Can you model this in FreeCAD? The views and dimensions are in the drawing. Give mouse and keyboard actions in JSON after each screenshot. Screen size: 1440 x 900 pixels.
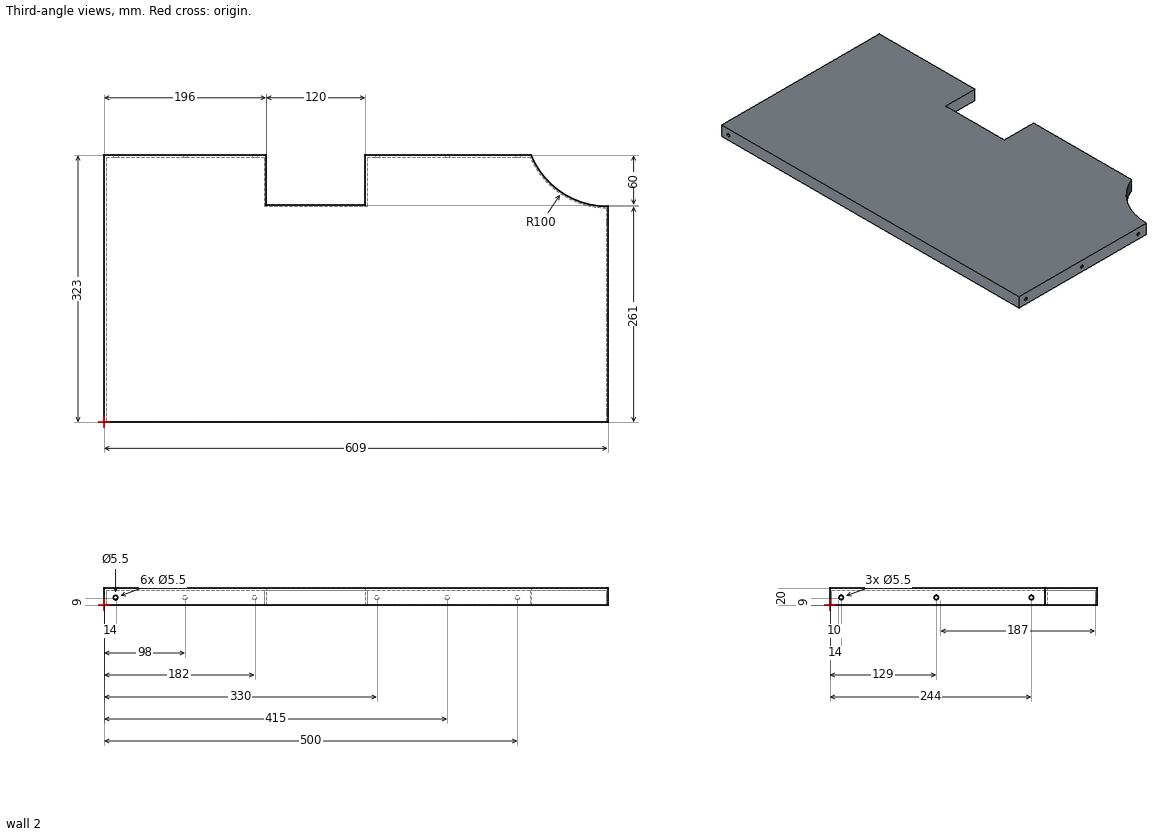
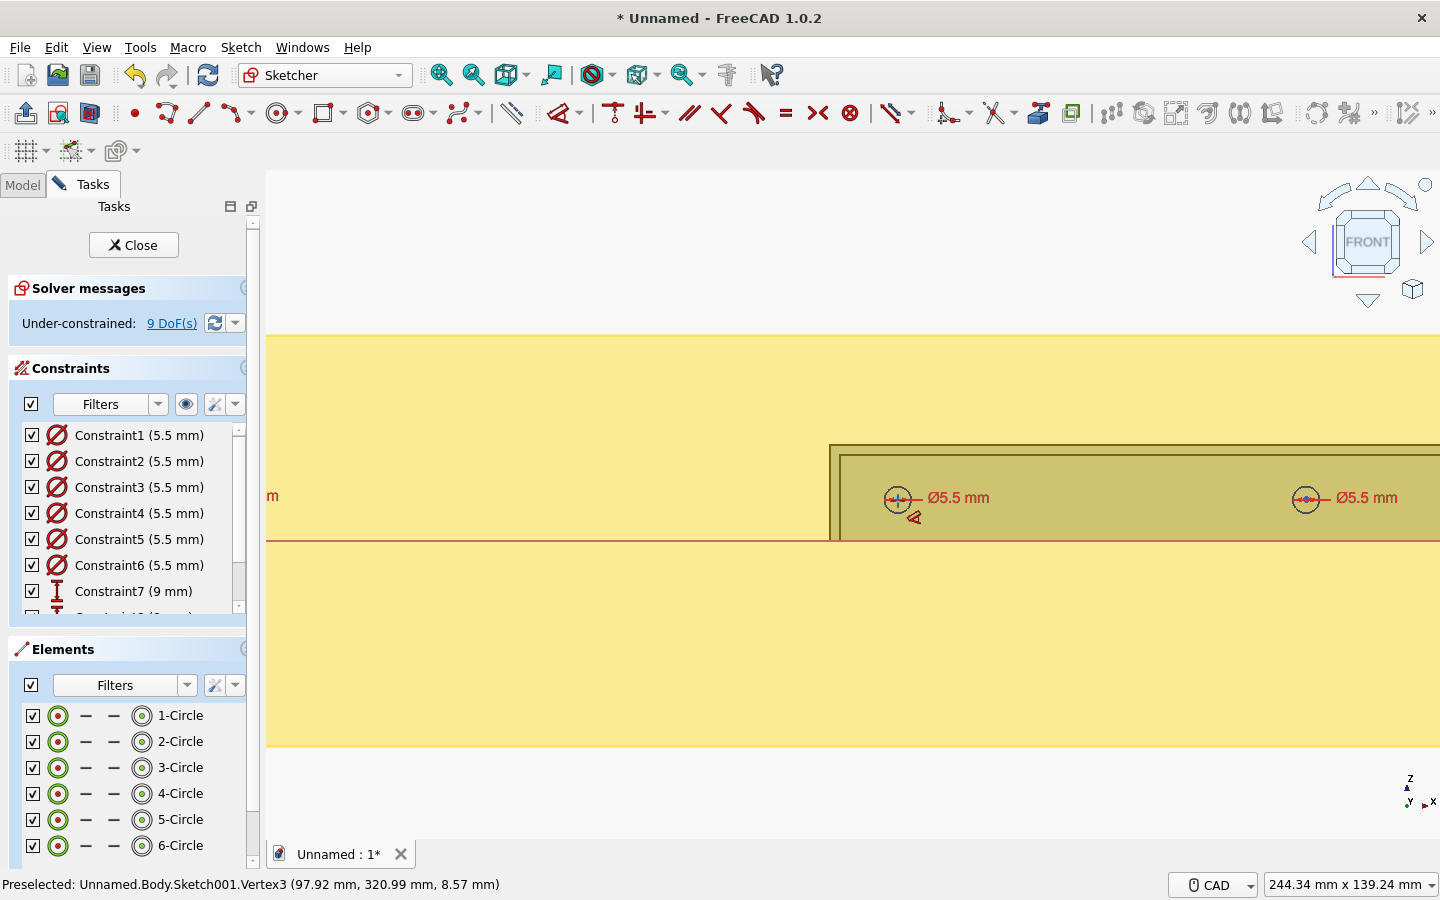
{"action": "left_click", "coordinate": [898, 500]}
{"action": "left_click", "coordinate": [932, 520]}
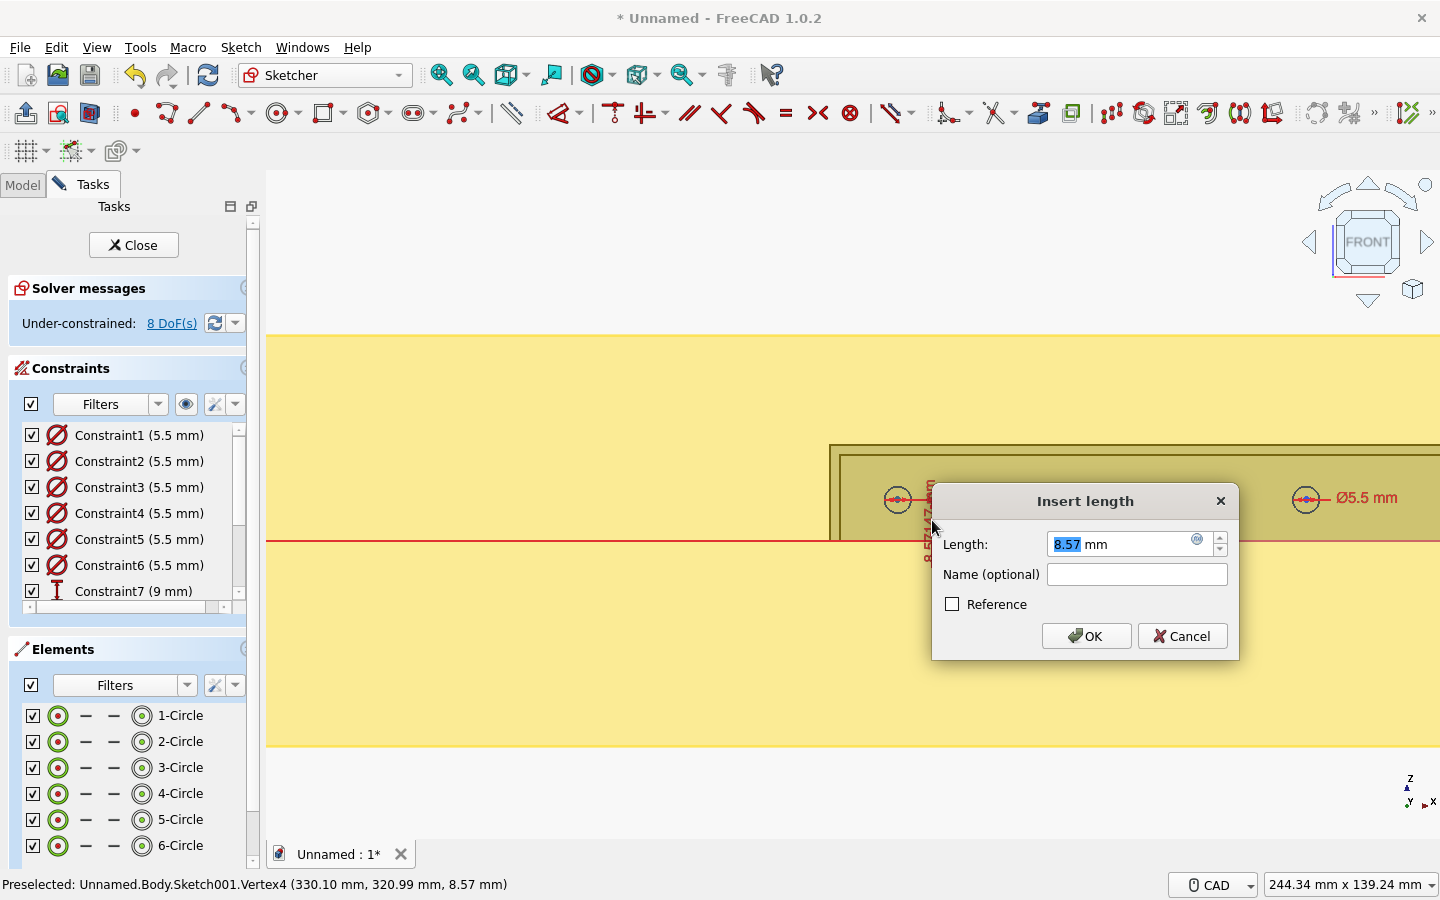
{"action": "type", "text": "9"}
{"action": "key", "text": "Return"}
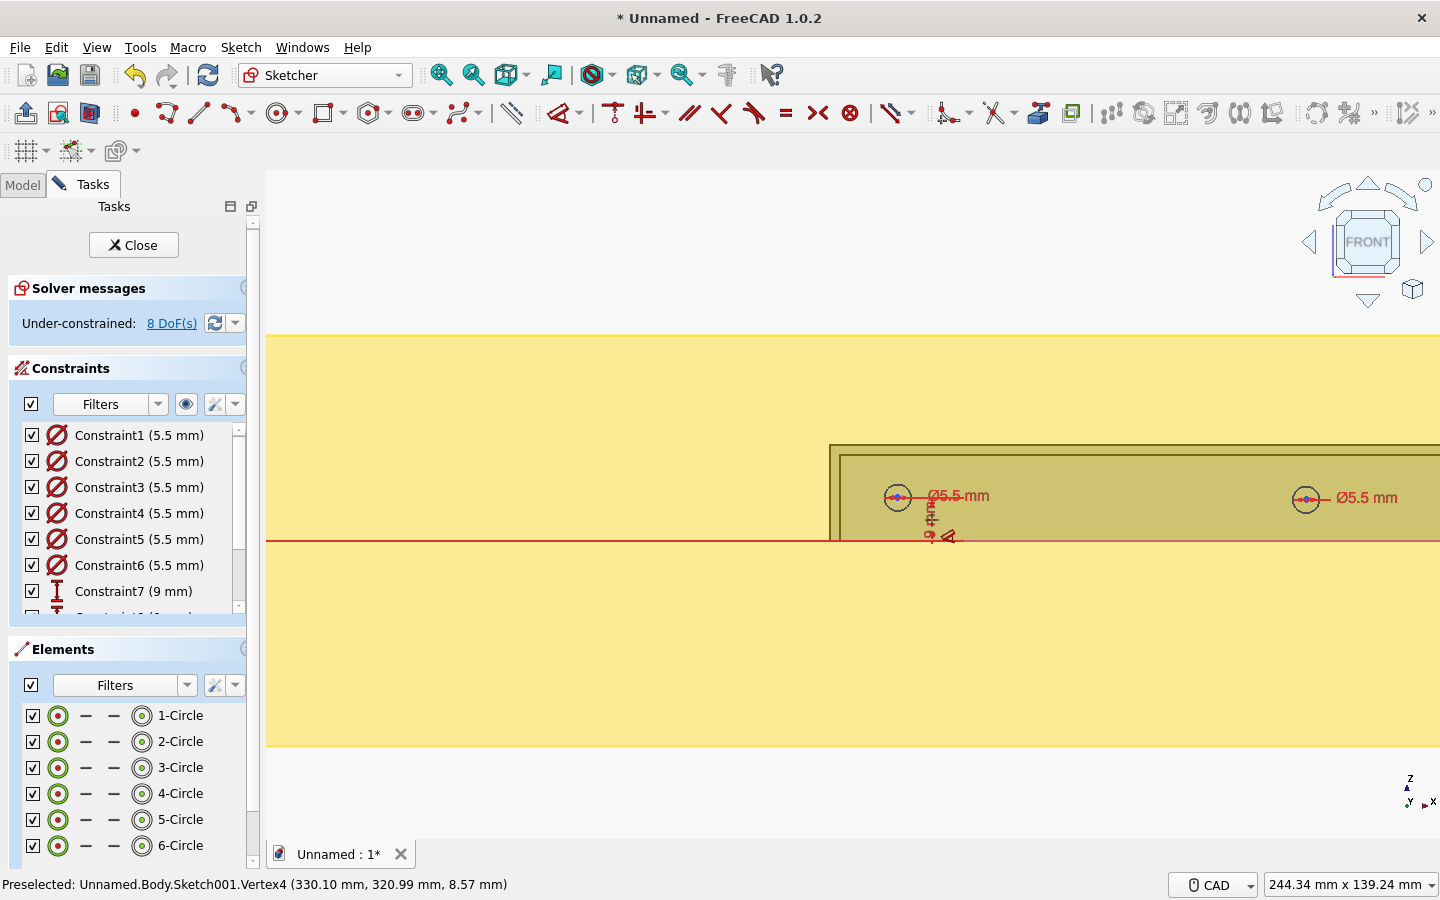
{"action": "scroll", "coordinate": [899, 501], "scroll_direction": "down", "scroll_amount": 6}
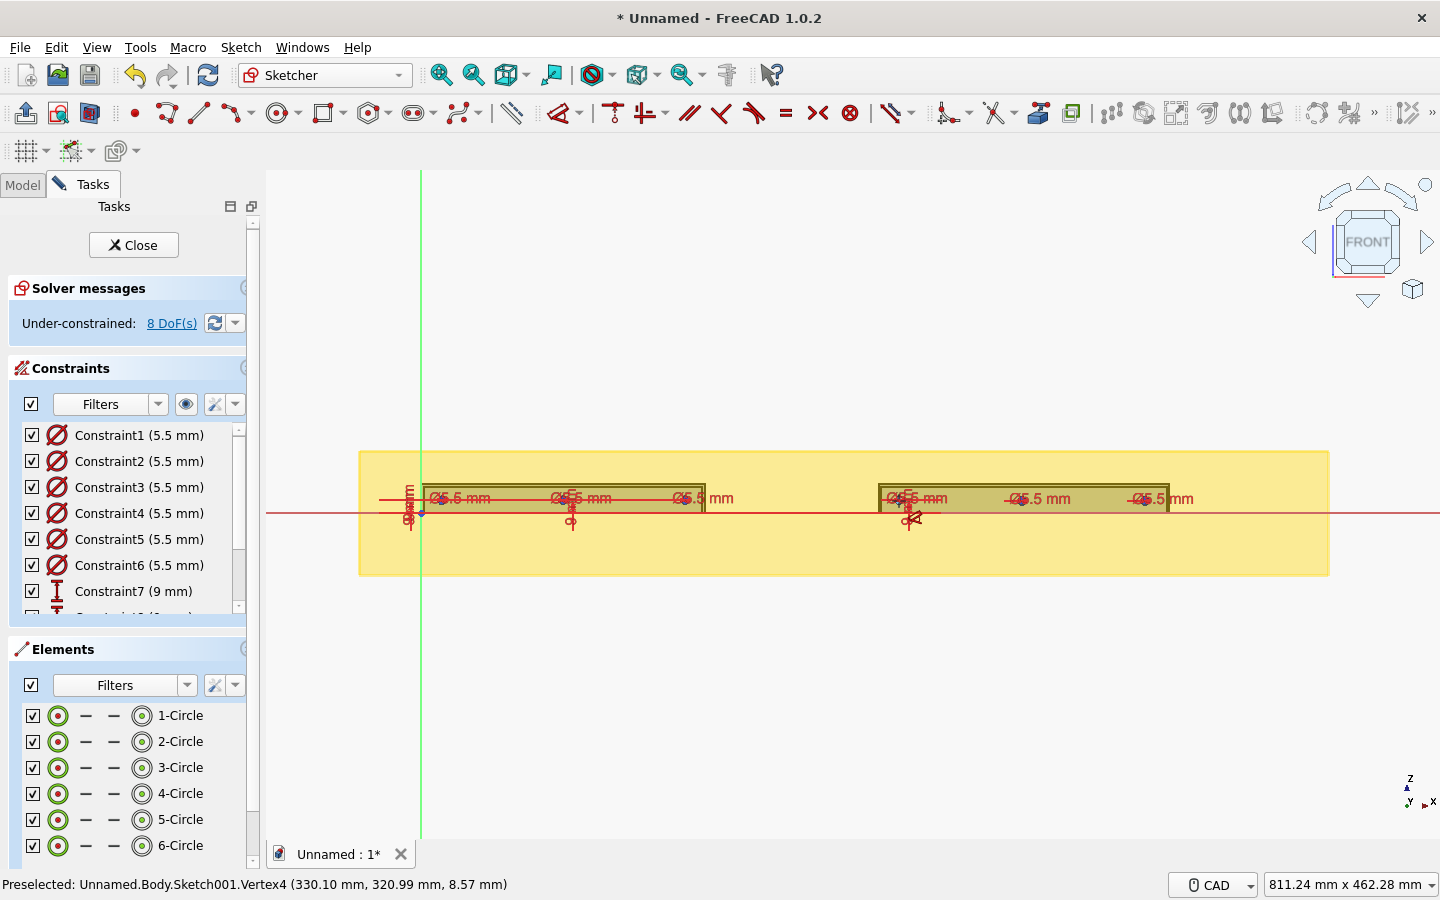
{"action": "scroll", "coordinate": [1145, 501], "scroll_direction": "up", "scroll_amount": 6}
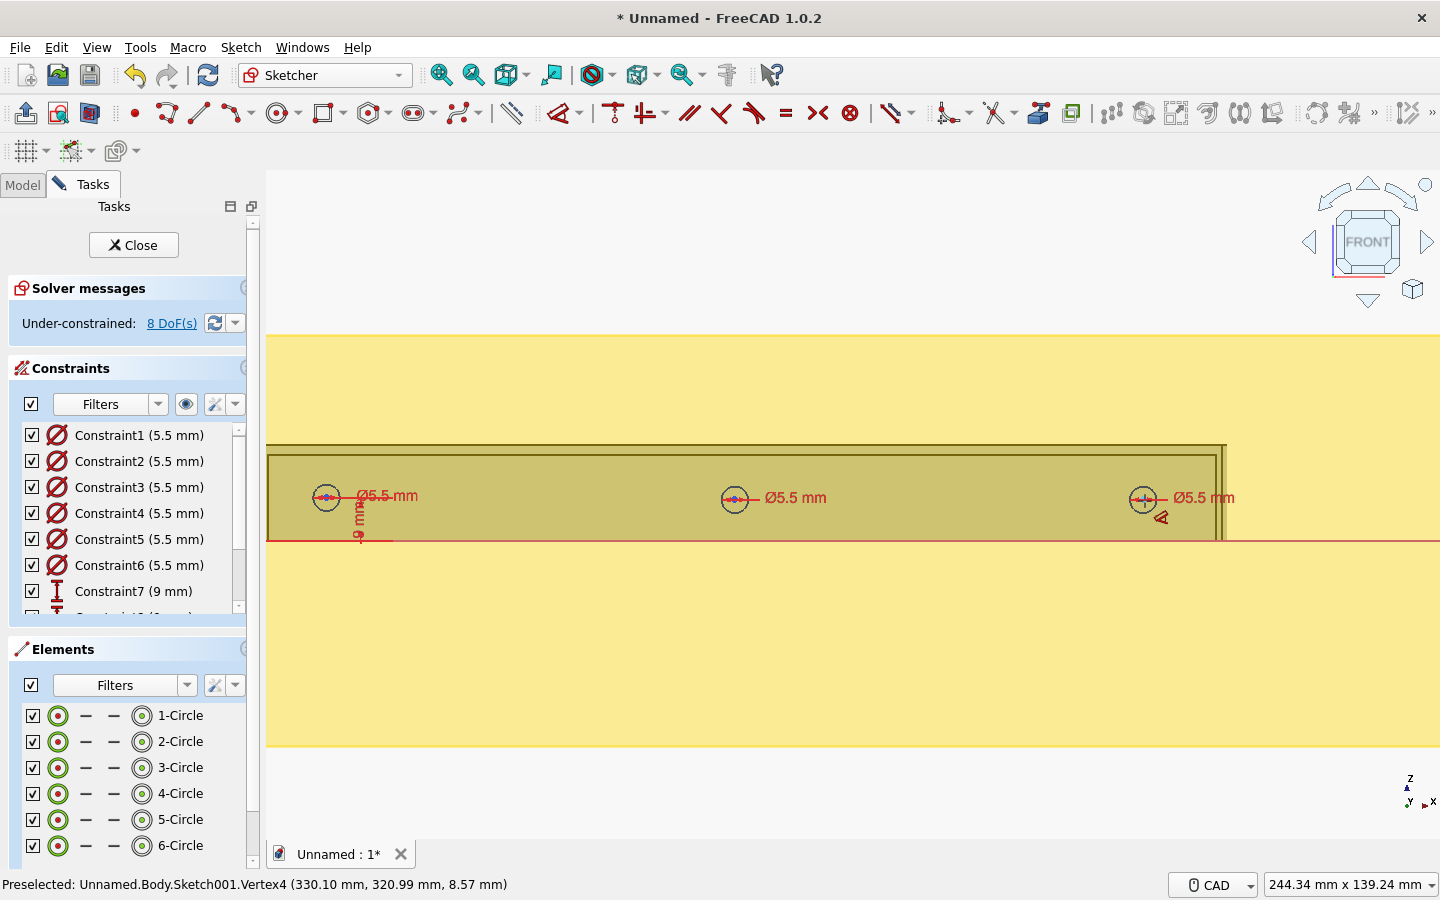
{"action": "left_click", "coordinate": [1143, 500]}
{"action": "left_click", "coordinate": [1177, 520]}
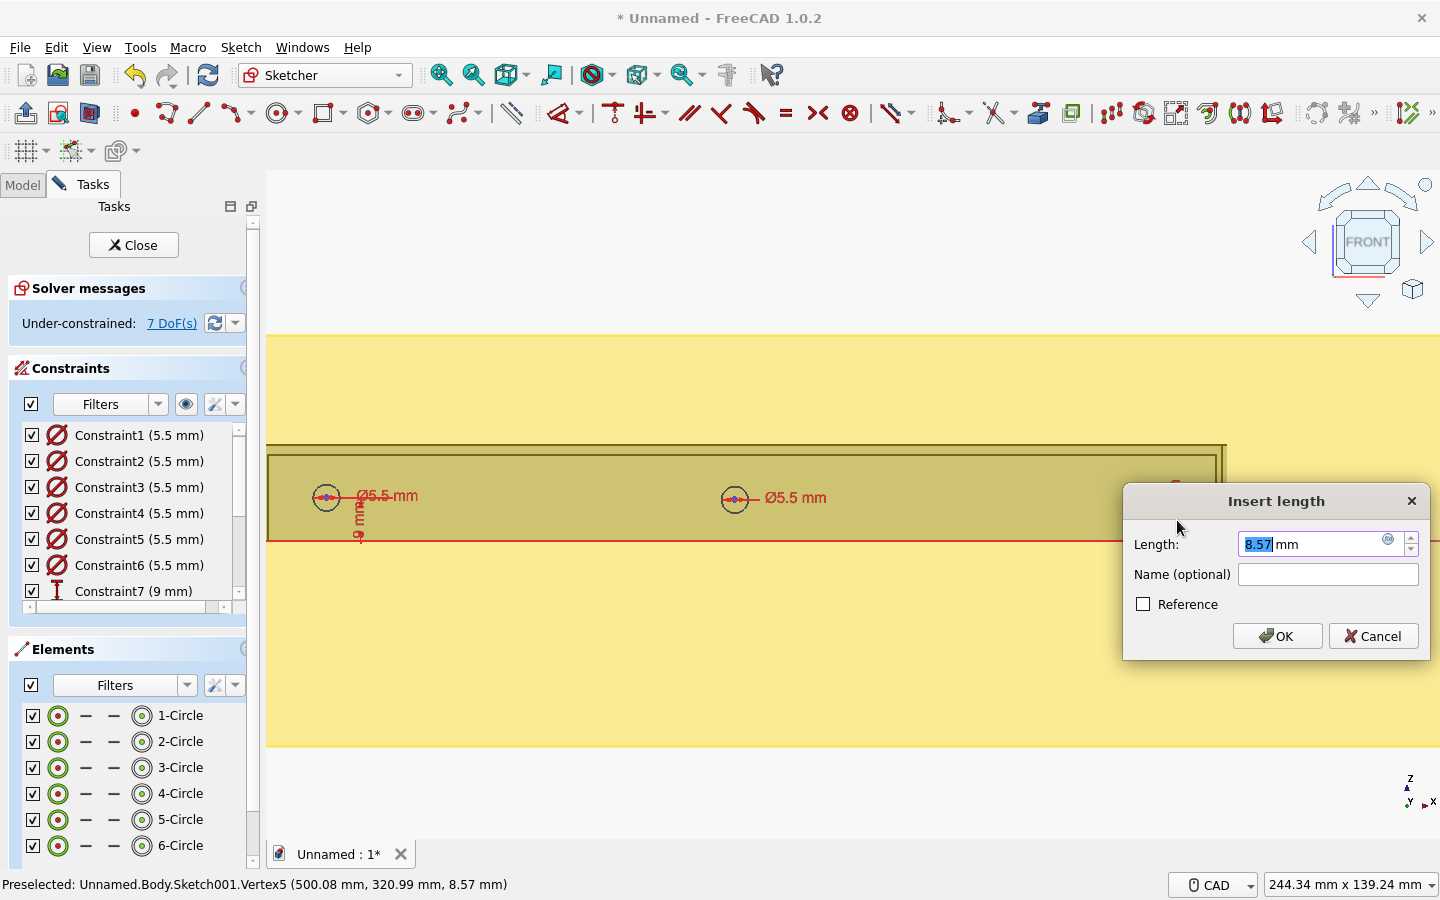
{"action": "type", "text": "9"}
{"action": "key", "text": "Return"}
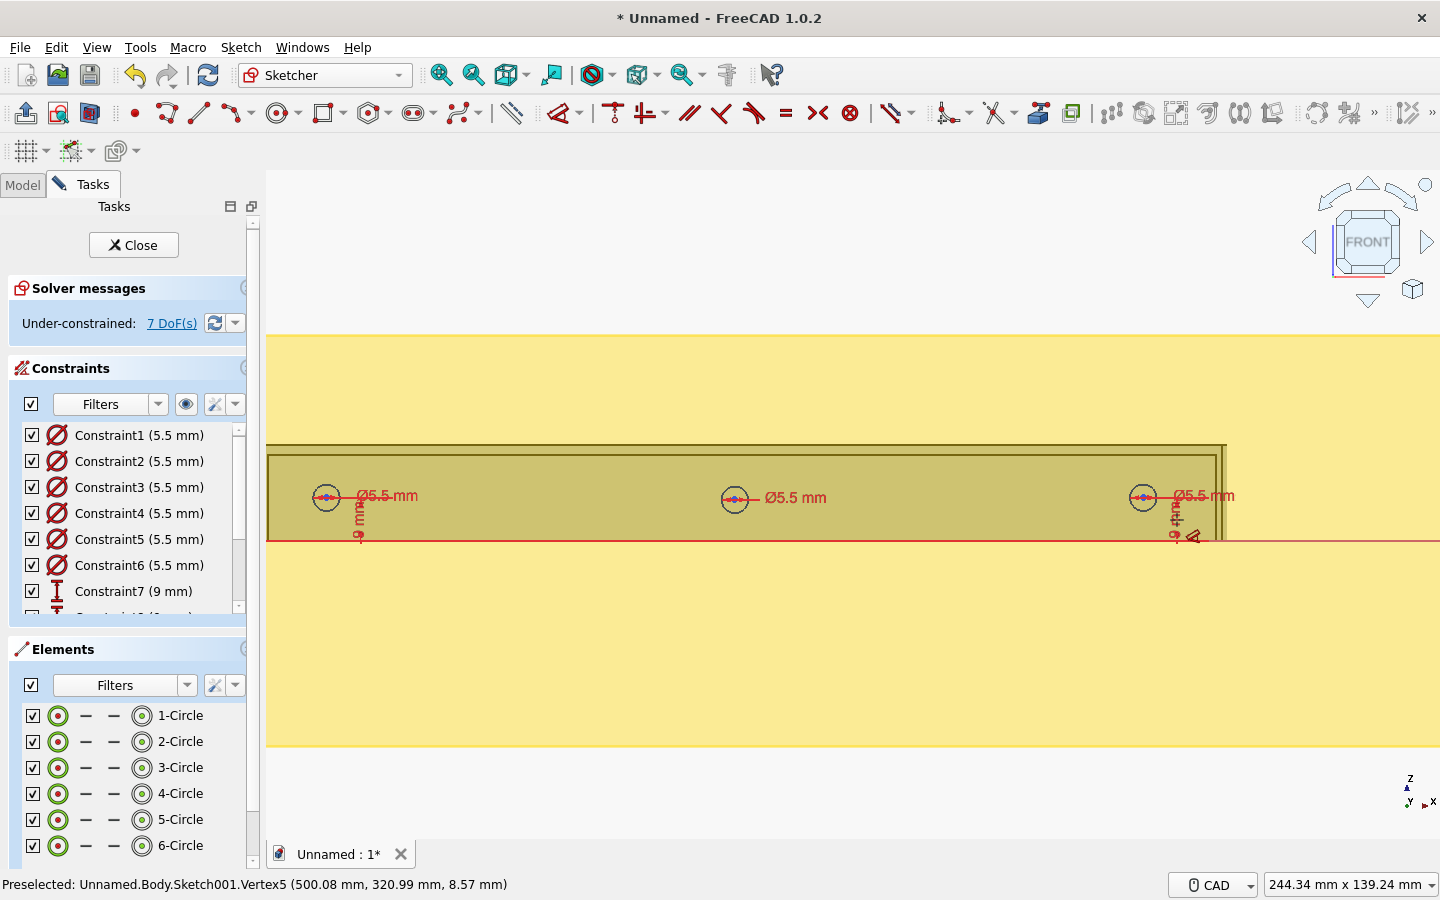
{"action": "left_click", "coordinate": [735, 500]}
{"action": "left_click", "coordinate": [769, 520]}